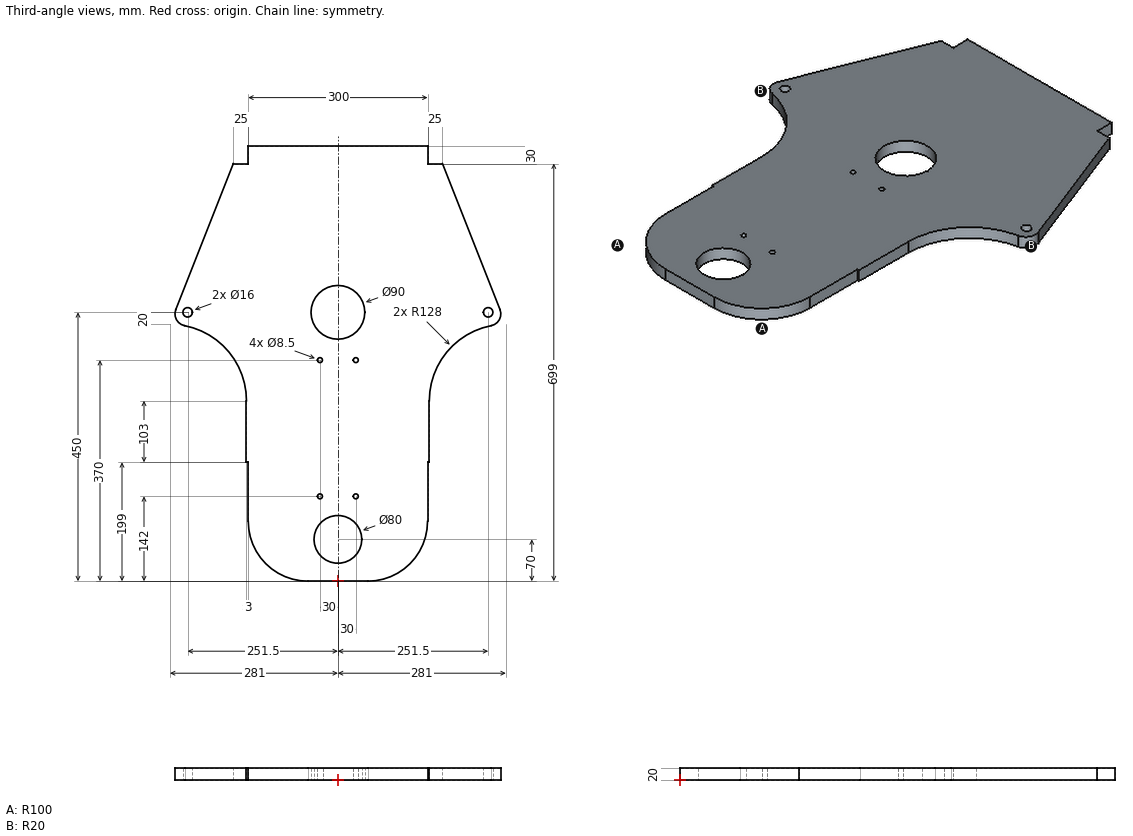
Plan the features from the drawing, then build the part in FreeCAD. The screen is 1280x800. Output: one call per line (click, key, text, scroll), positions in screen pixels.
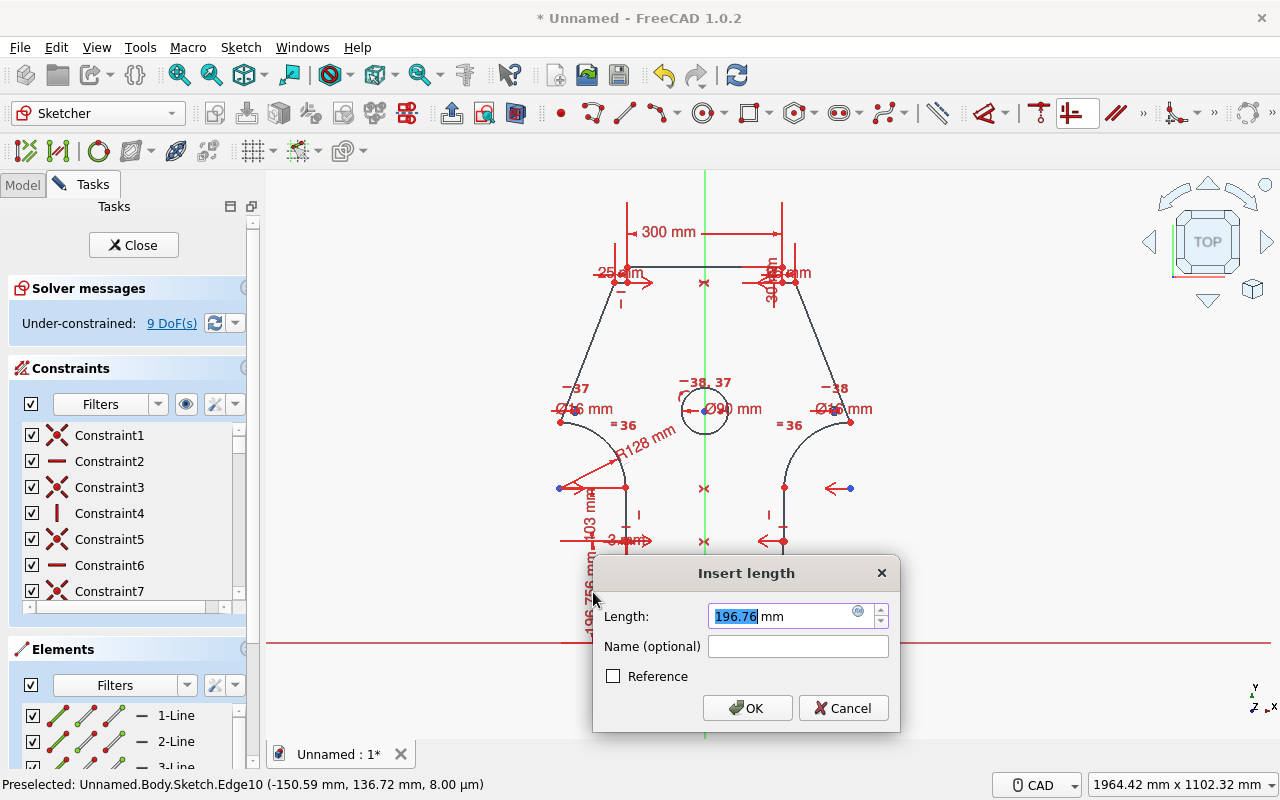
text(199)
key(Return)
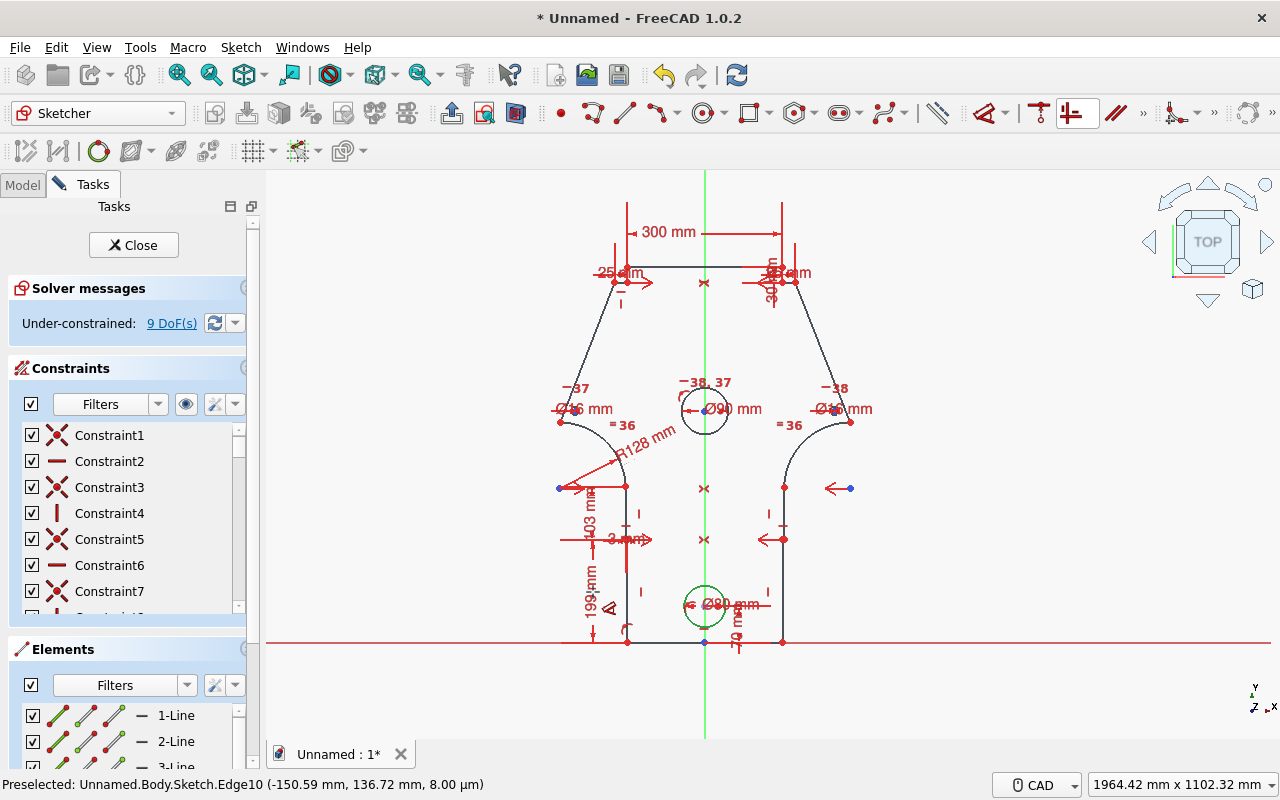
click(674, 643)
click(669, 677)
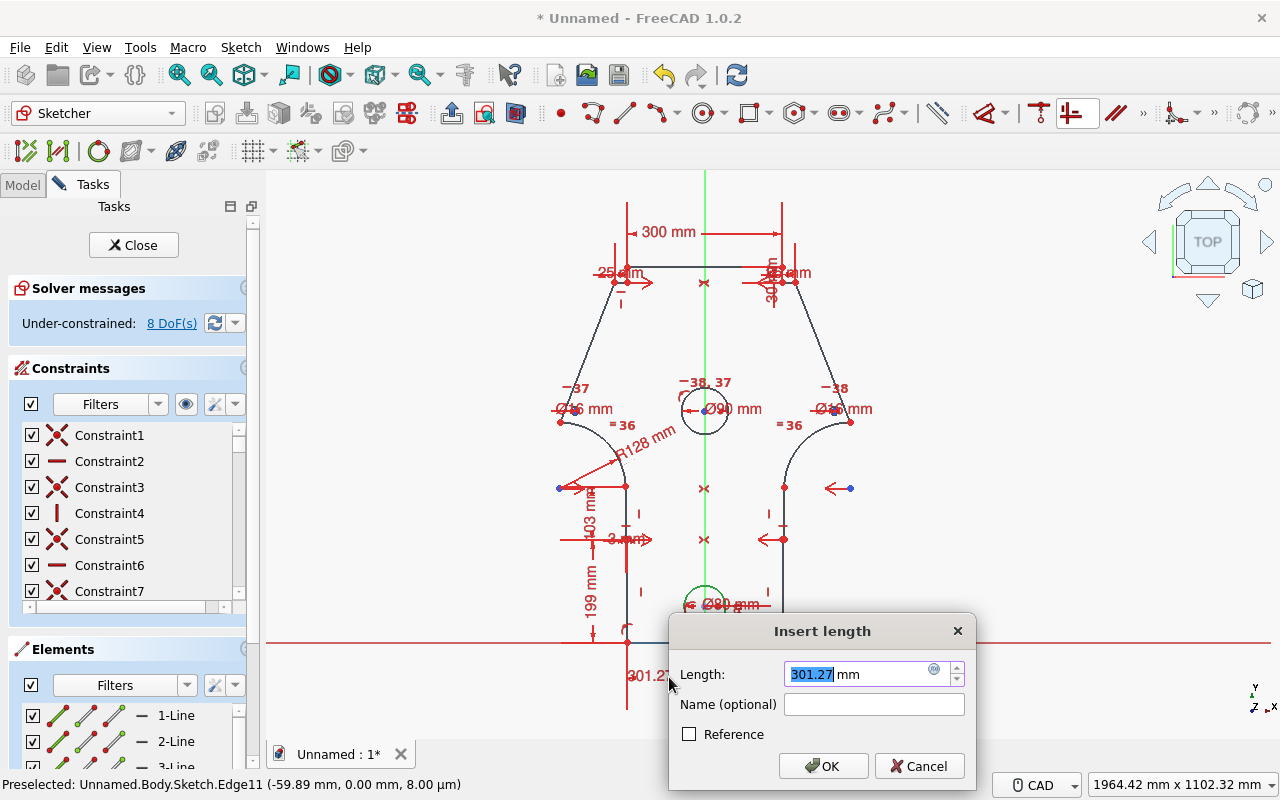
text(300)
key(Return)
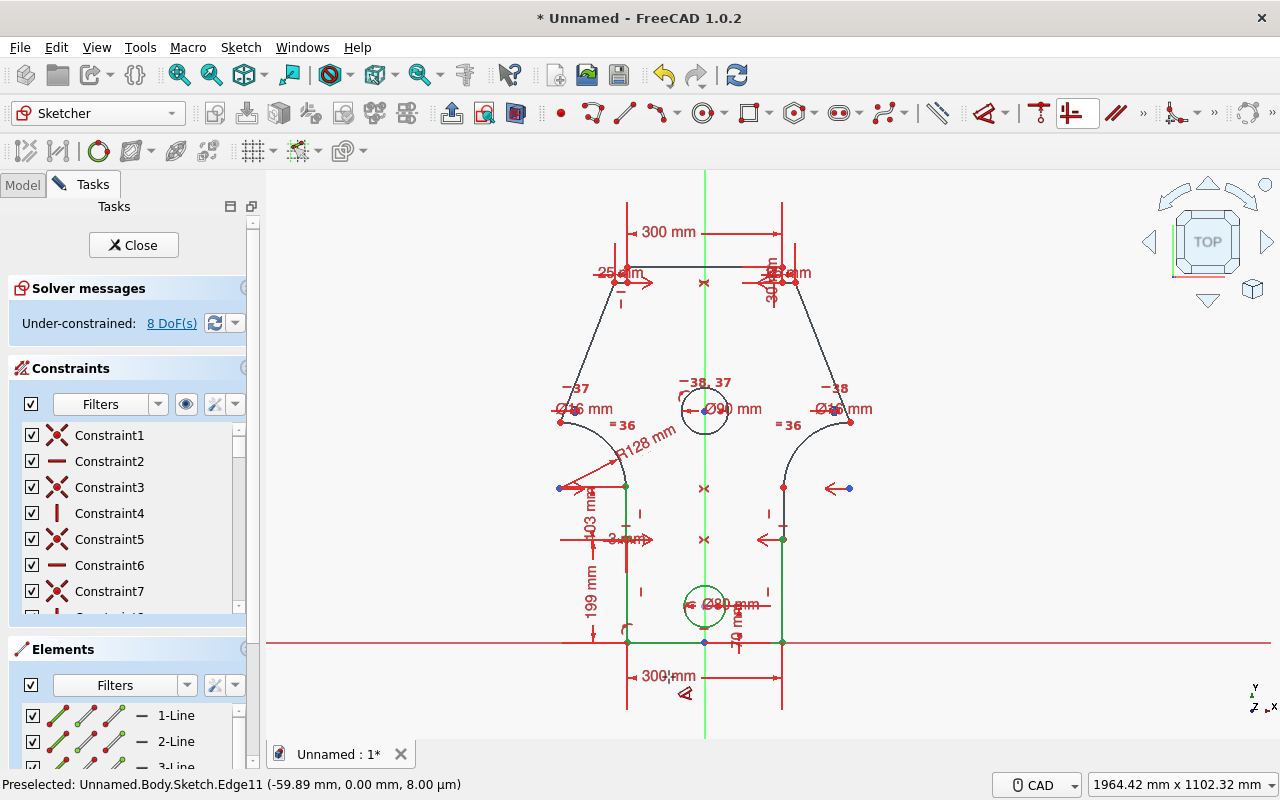
click(784, 524)
click(818, 514)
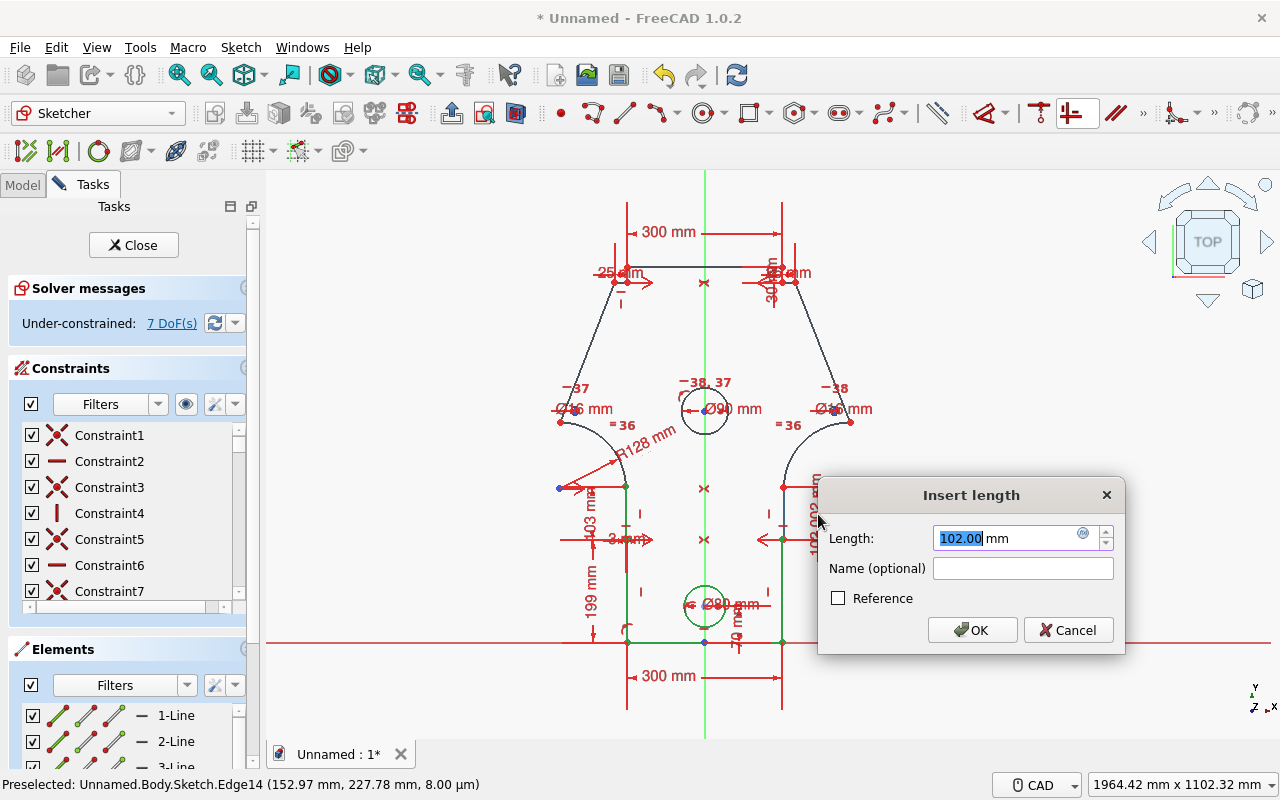
text(103)
key(Return)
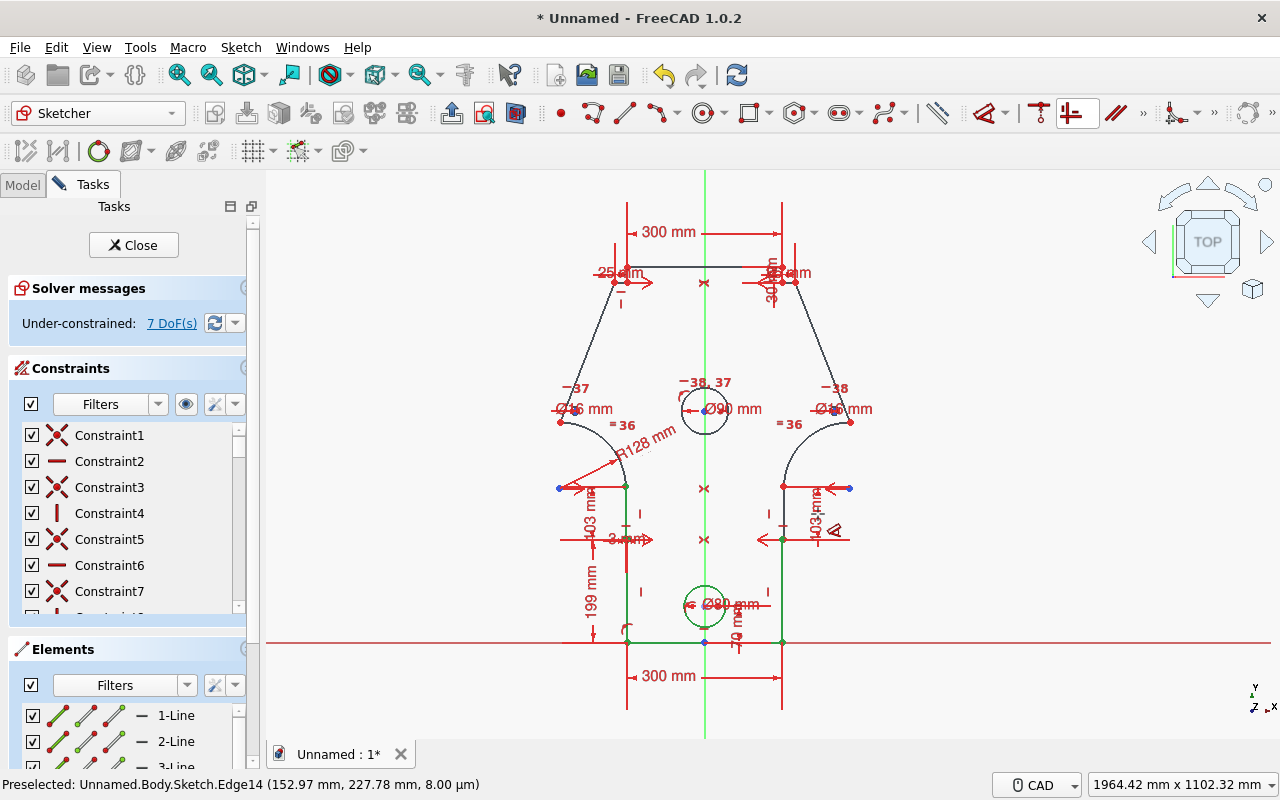
click(575, 411)
click(541, 474)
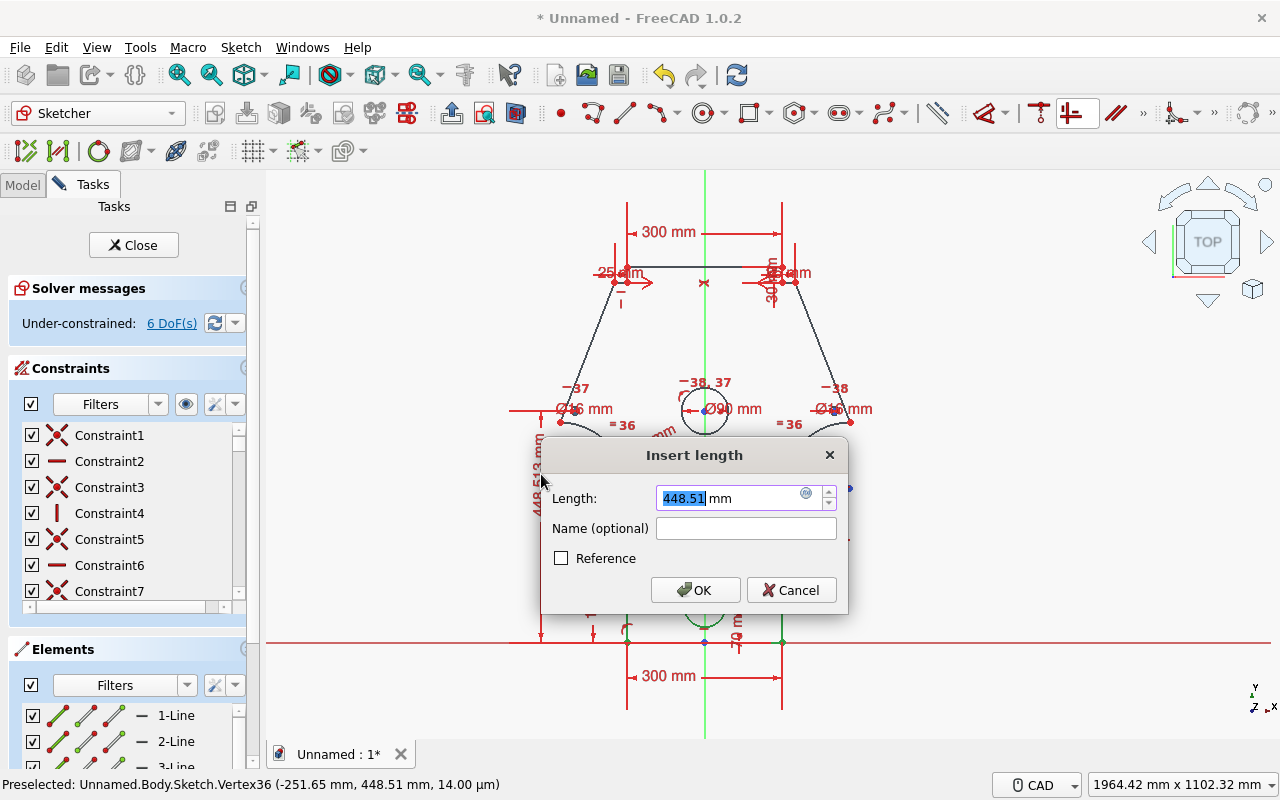
text(450)
key(Return)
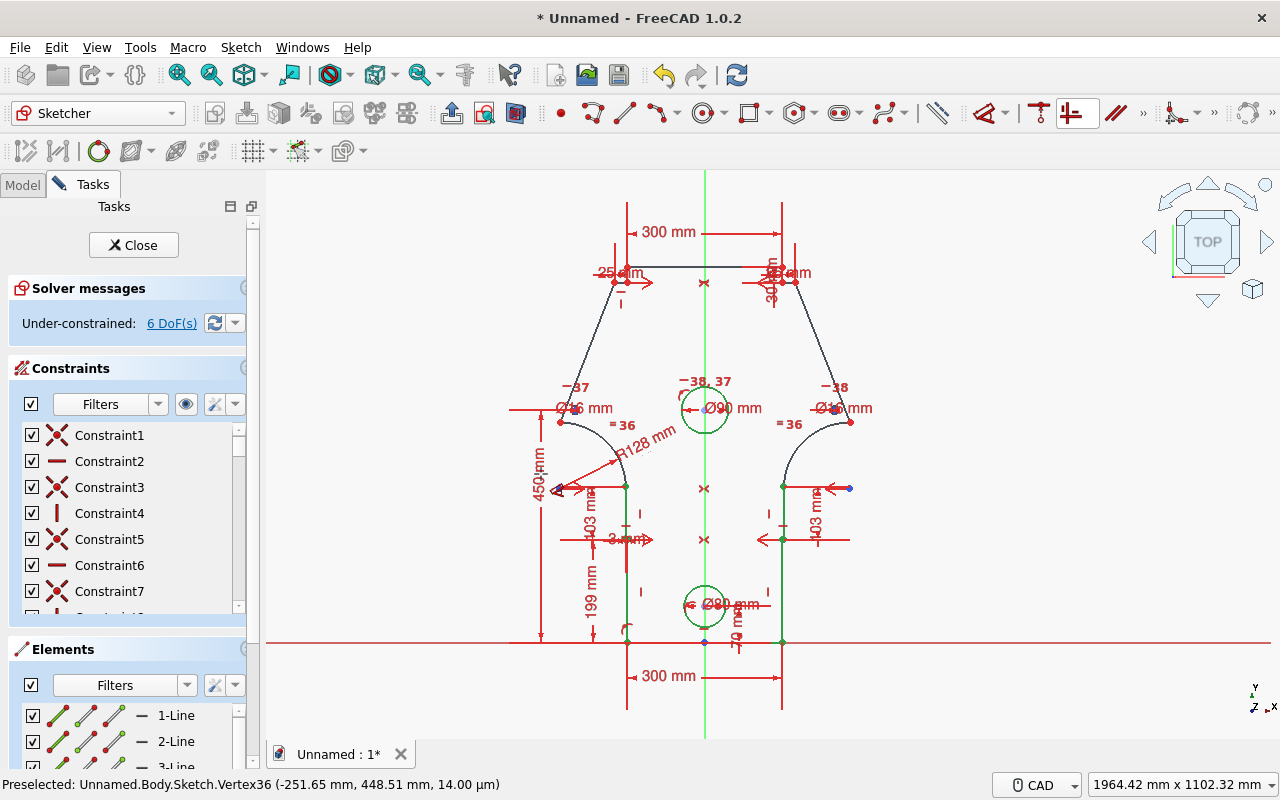
scroll(560, 423, up, 7)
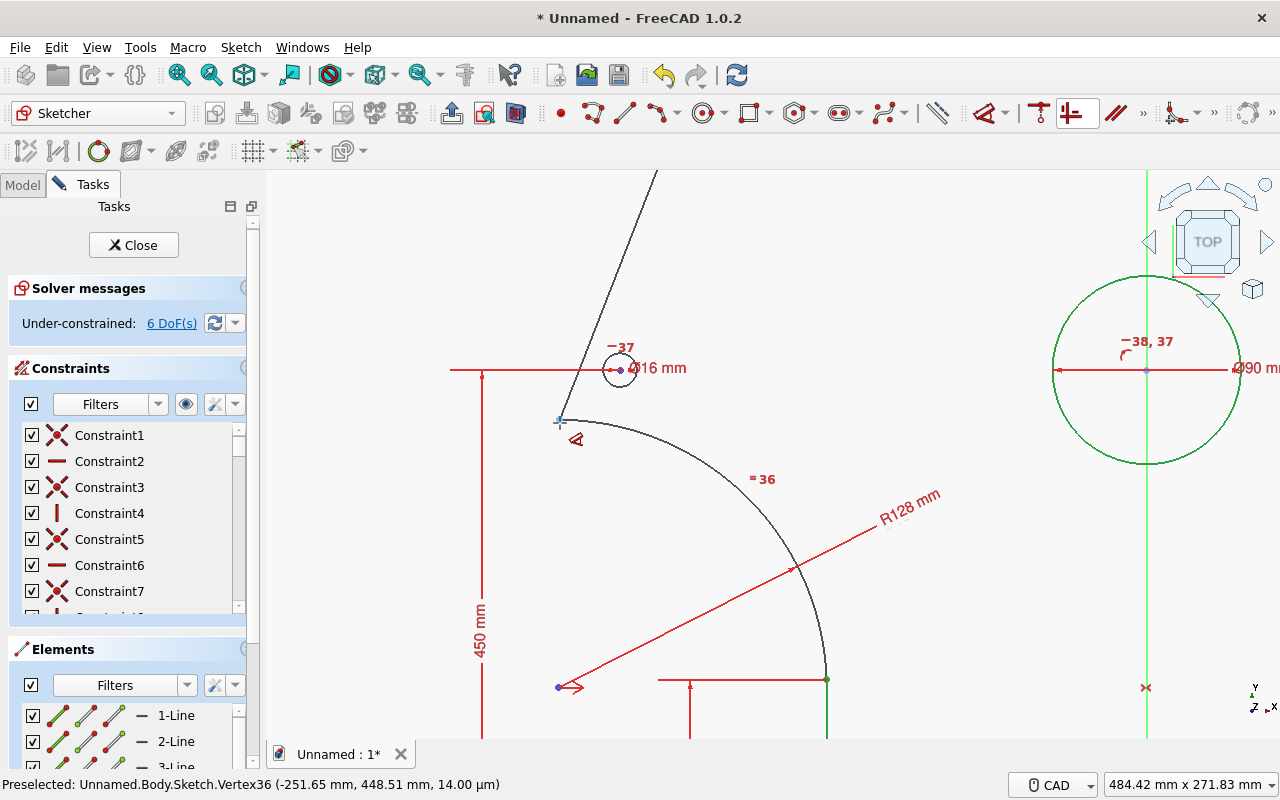
click(560, 420)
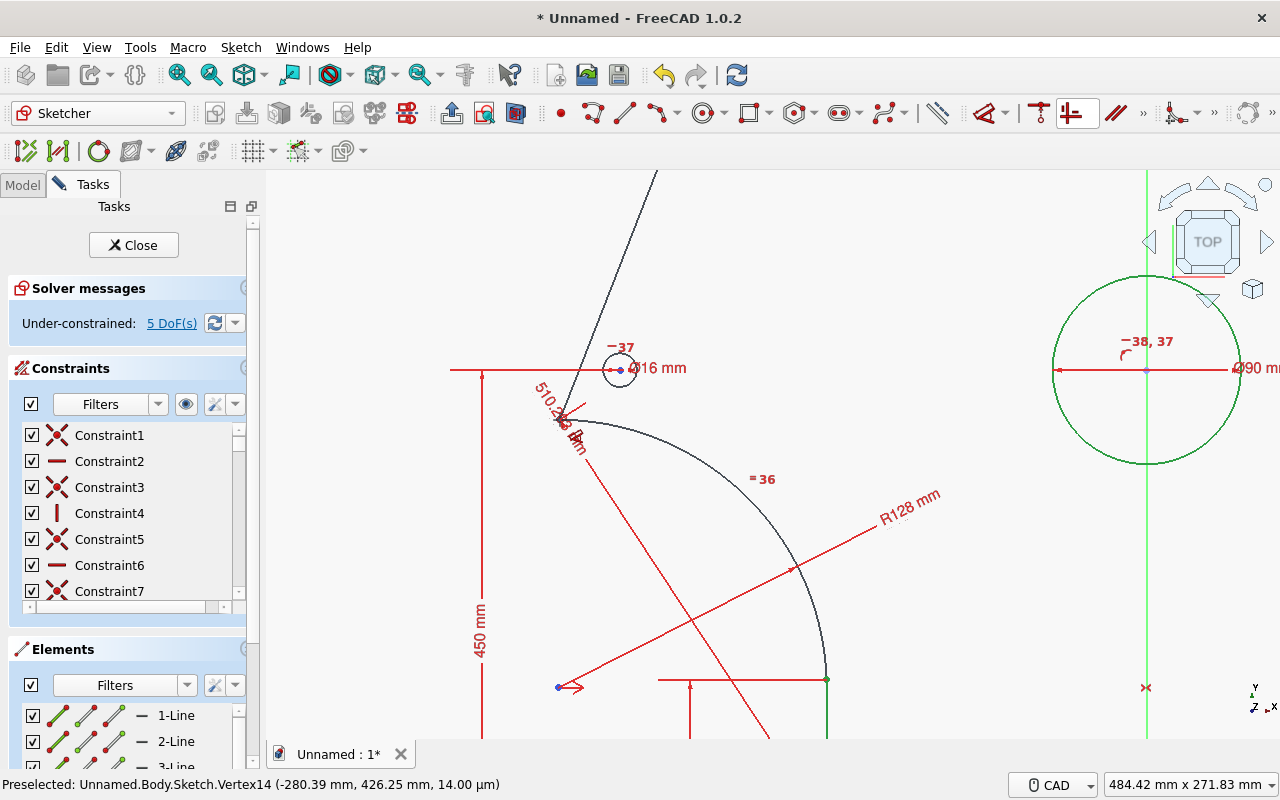
click(620, 370)
click(526, 395)